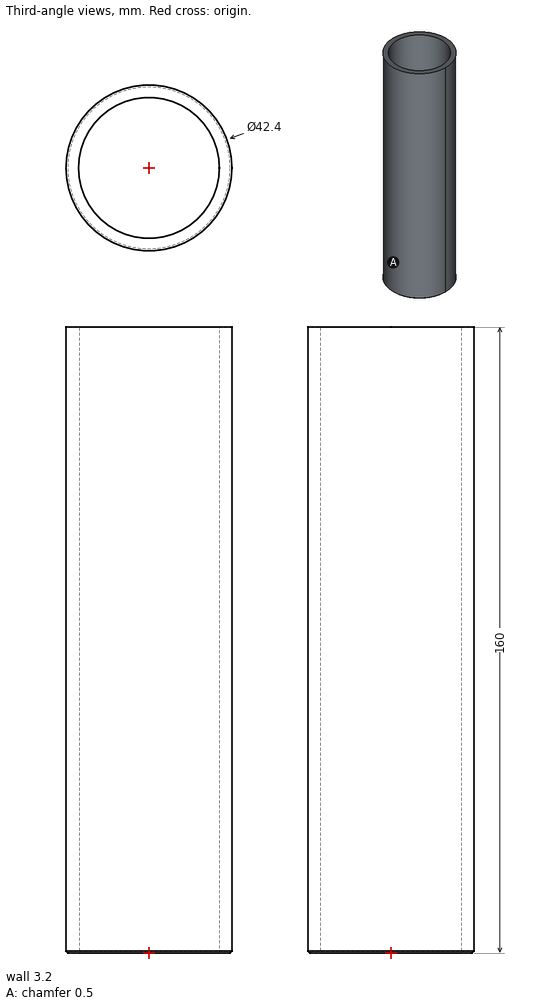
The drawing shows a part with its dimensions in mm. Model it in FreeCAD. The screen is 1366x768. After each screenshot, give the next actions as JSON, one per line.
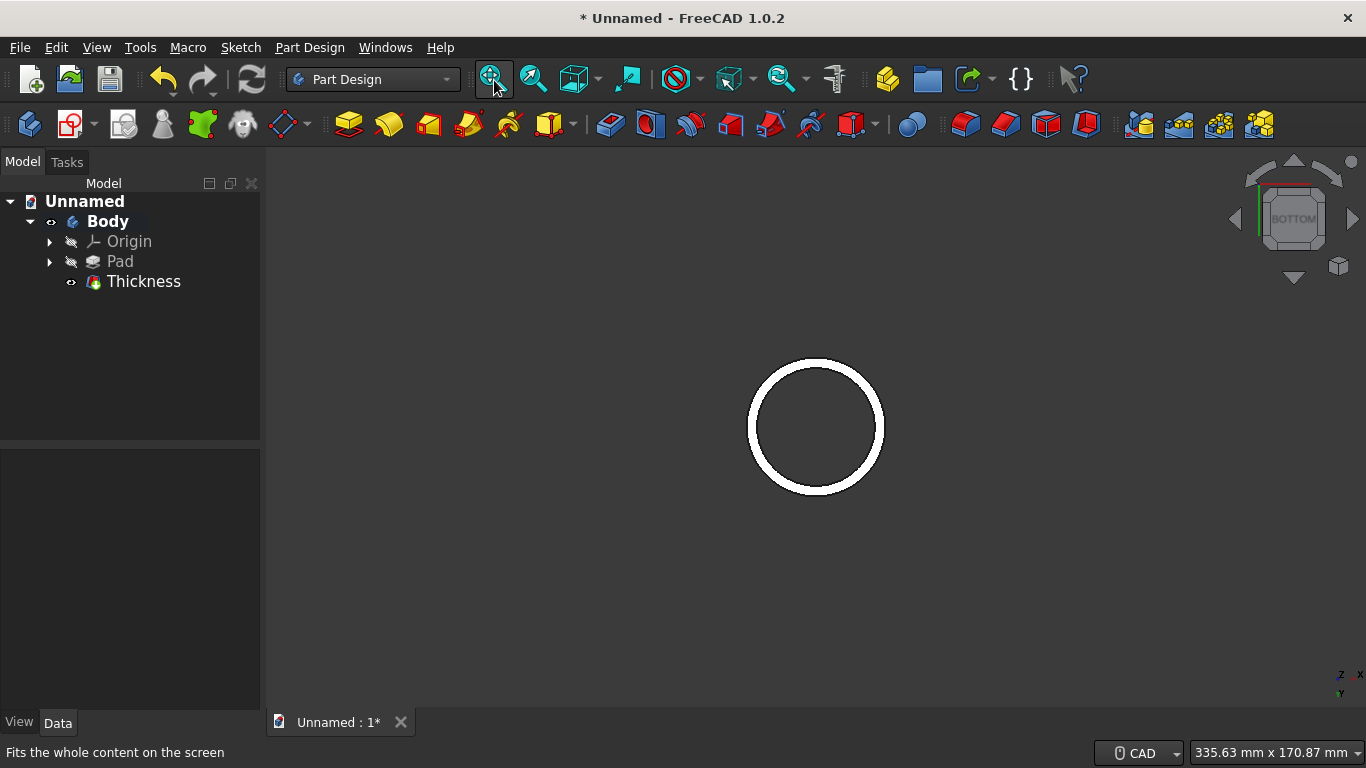
{"action": "left_click", "coordinate": [747, 426]}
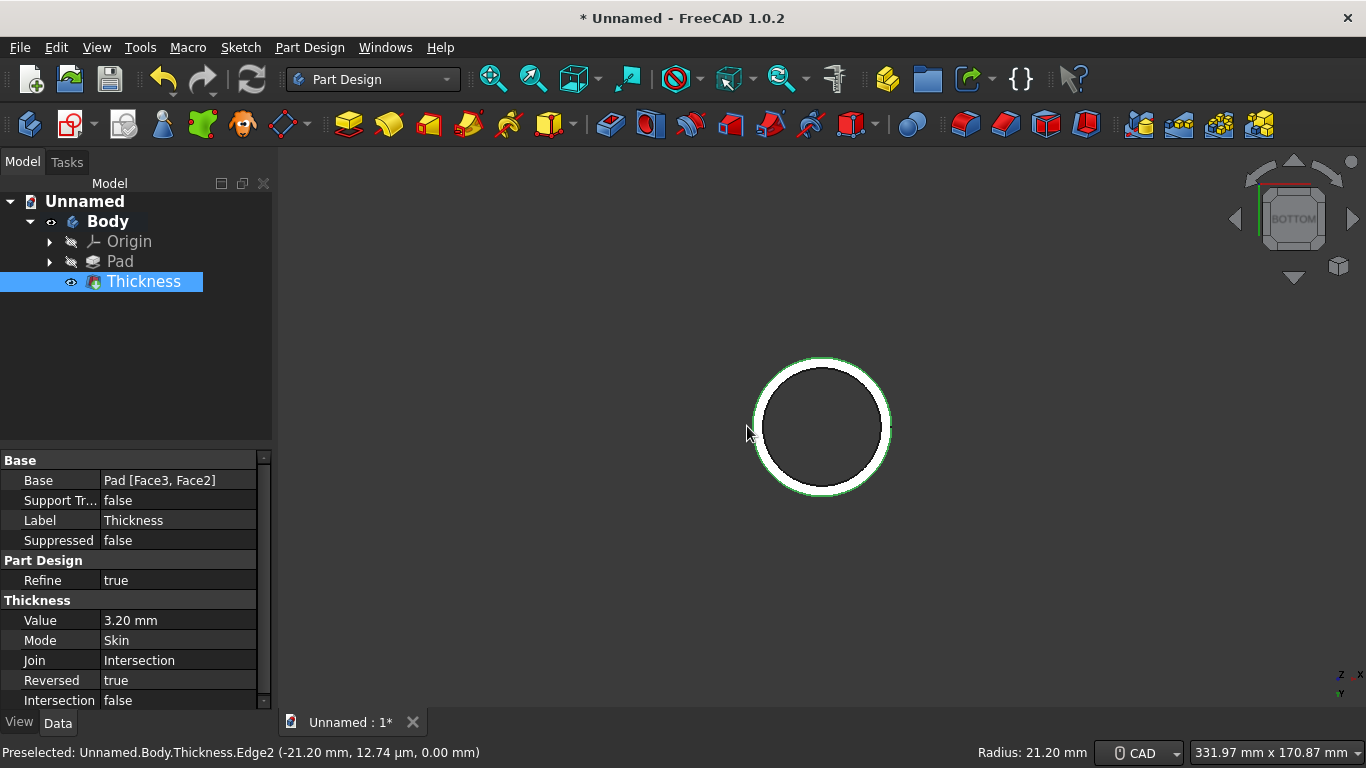
{"action": "left_click", "coordinate": [1006, 124]}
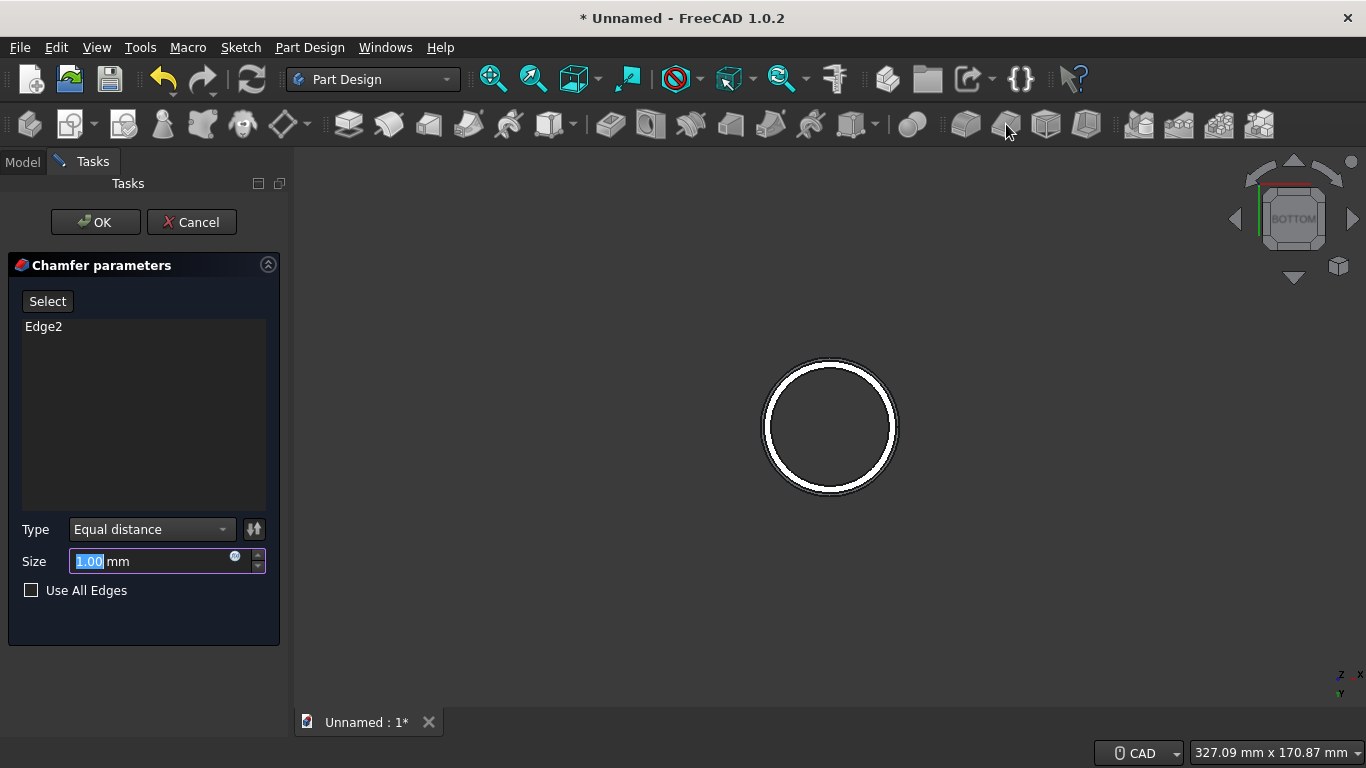
{"action": "type", "text": "0.5"}
{"action": "key", "text": "Tab"}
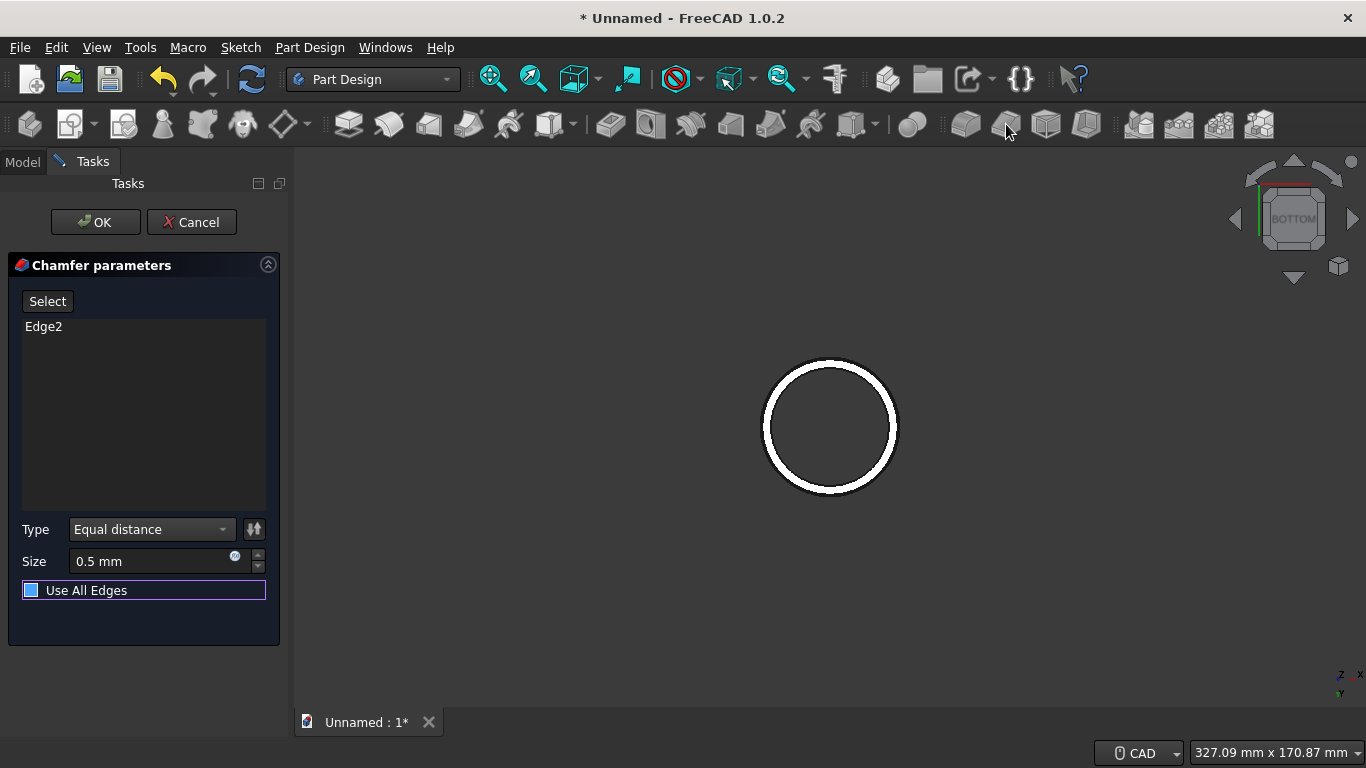
{"action": "left_click", "coordinate": [96, 222]}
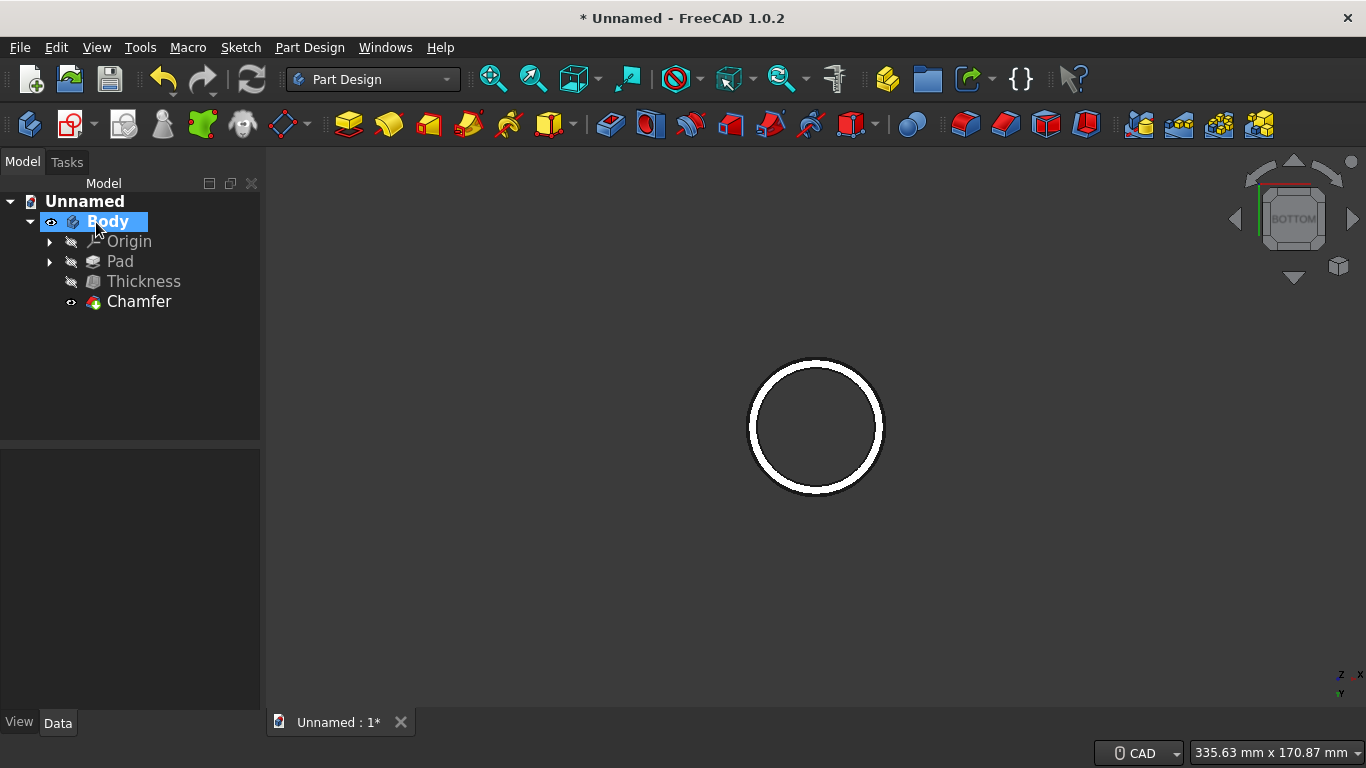
{"action": "key", "text": "0"}